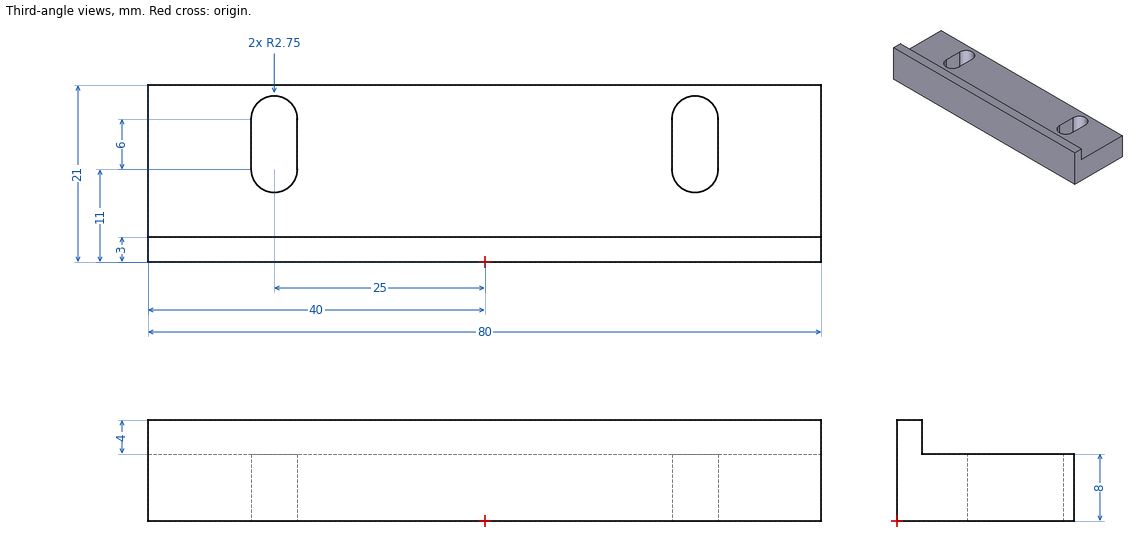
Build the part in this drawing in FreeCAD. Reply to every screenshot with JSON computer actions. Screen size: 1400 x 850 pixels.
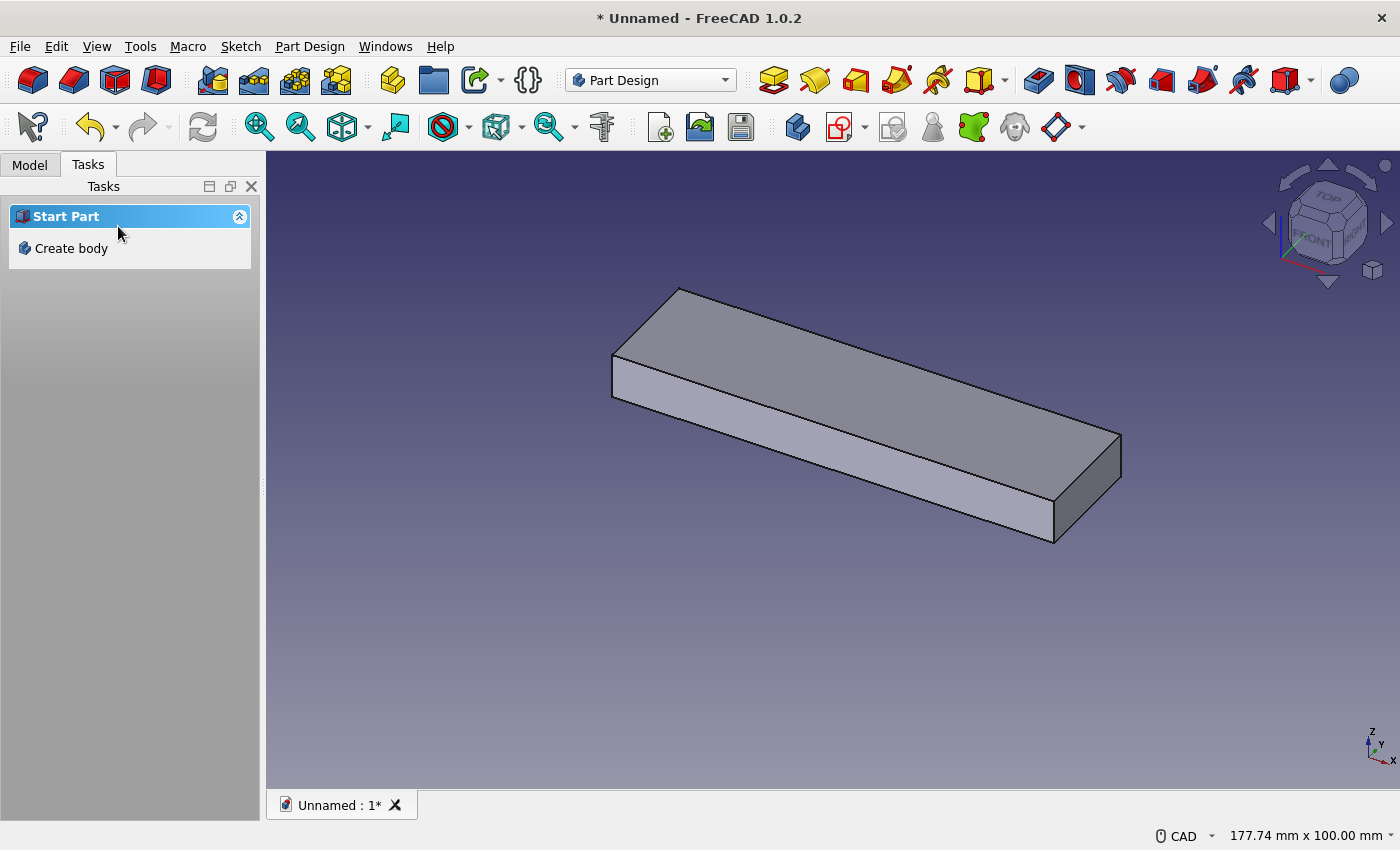
{"action": "key", "text": "v f"}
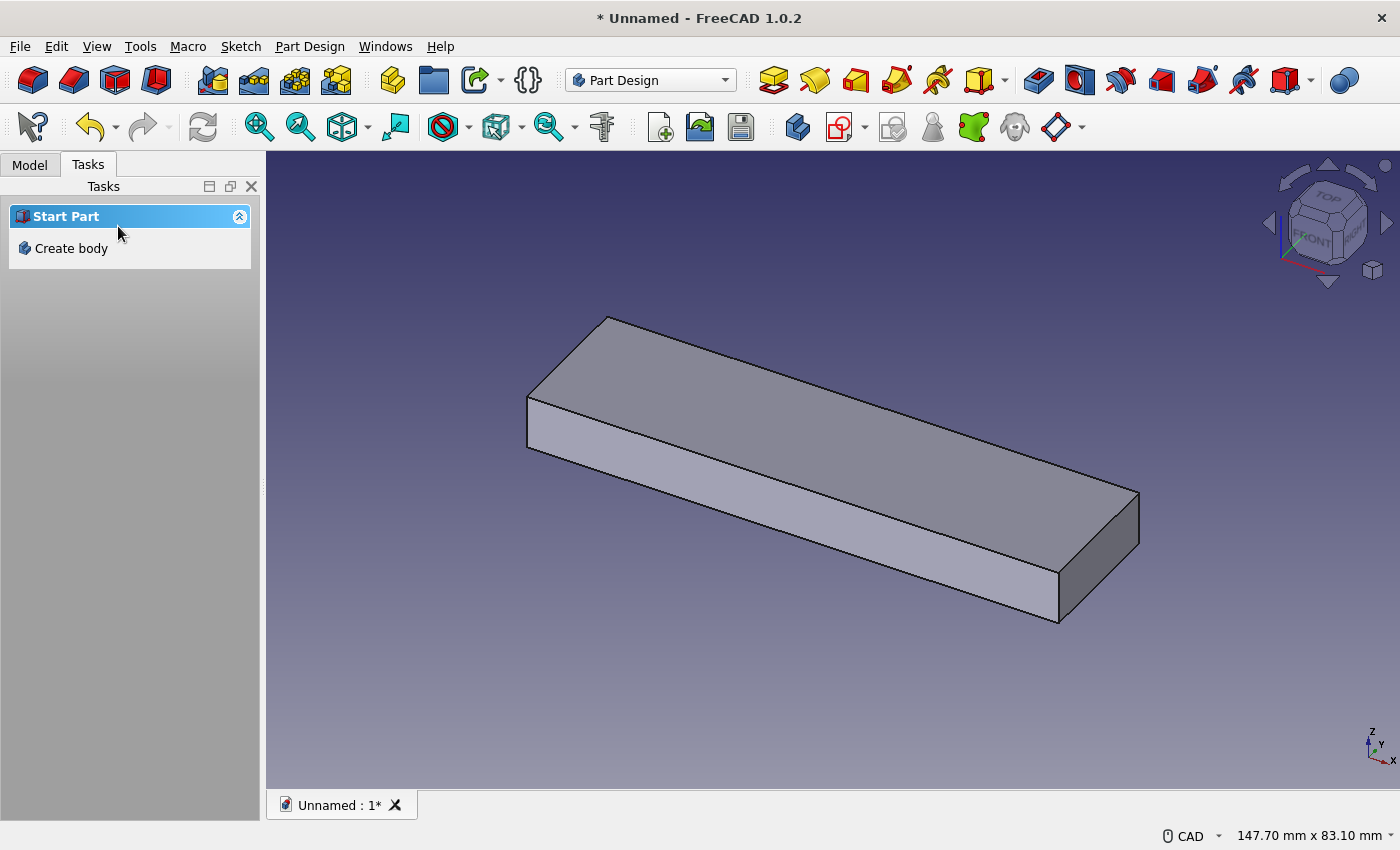
{"action": "left_click", "coordinate": [985, 494]}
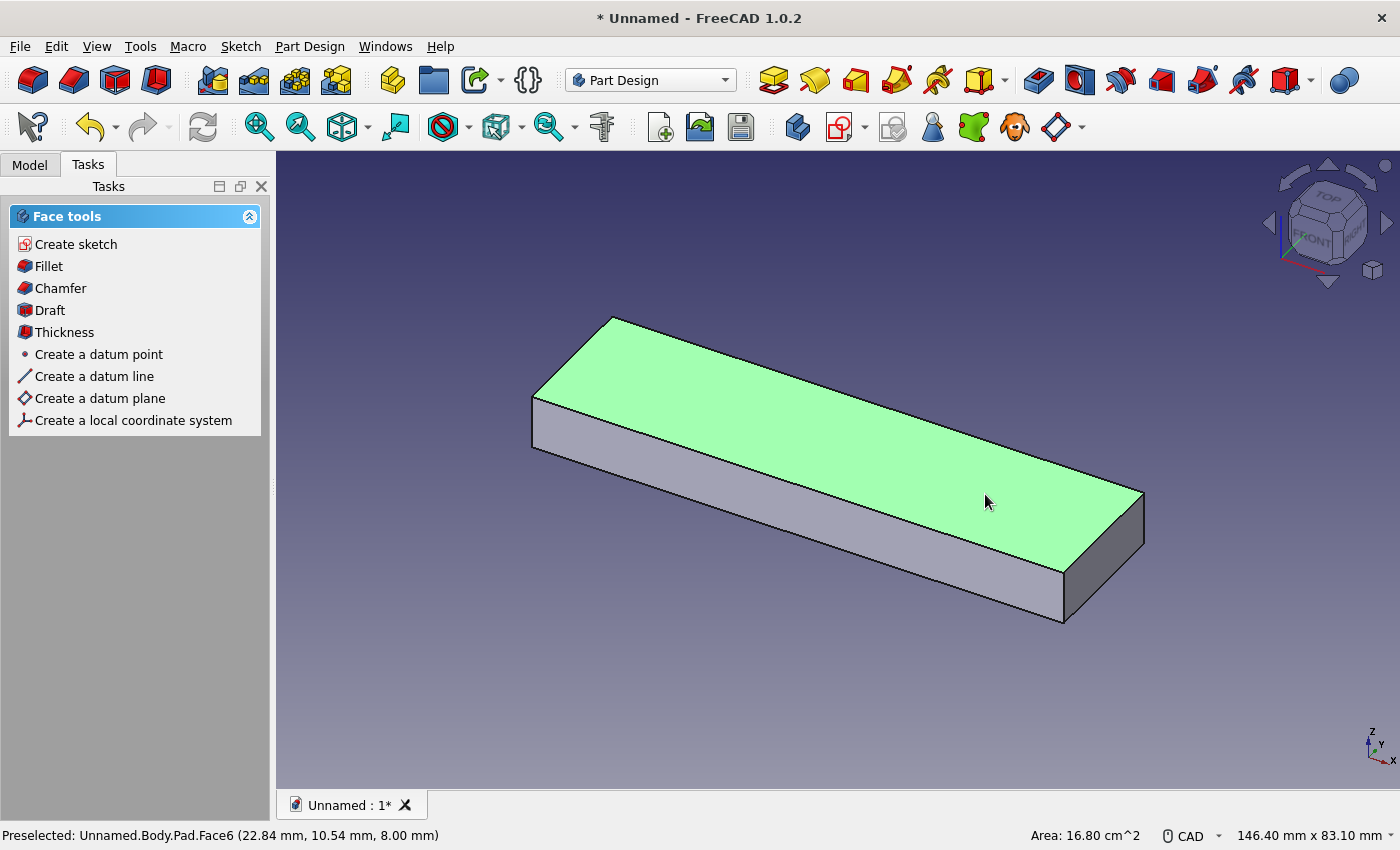
{"action": "left_click", "coordinate": [838, 128]}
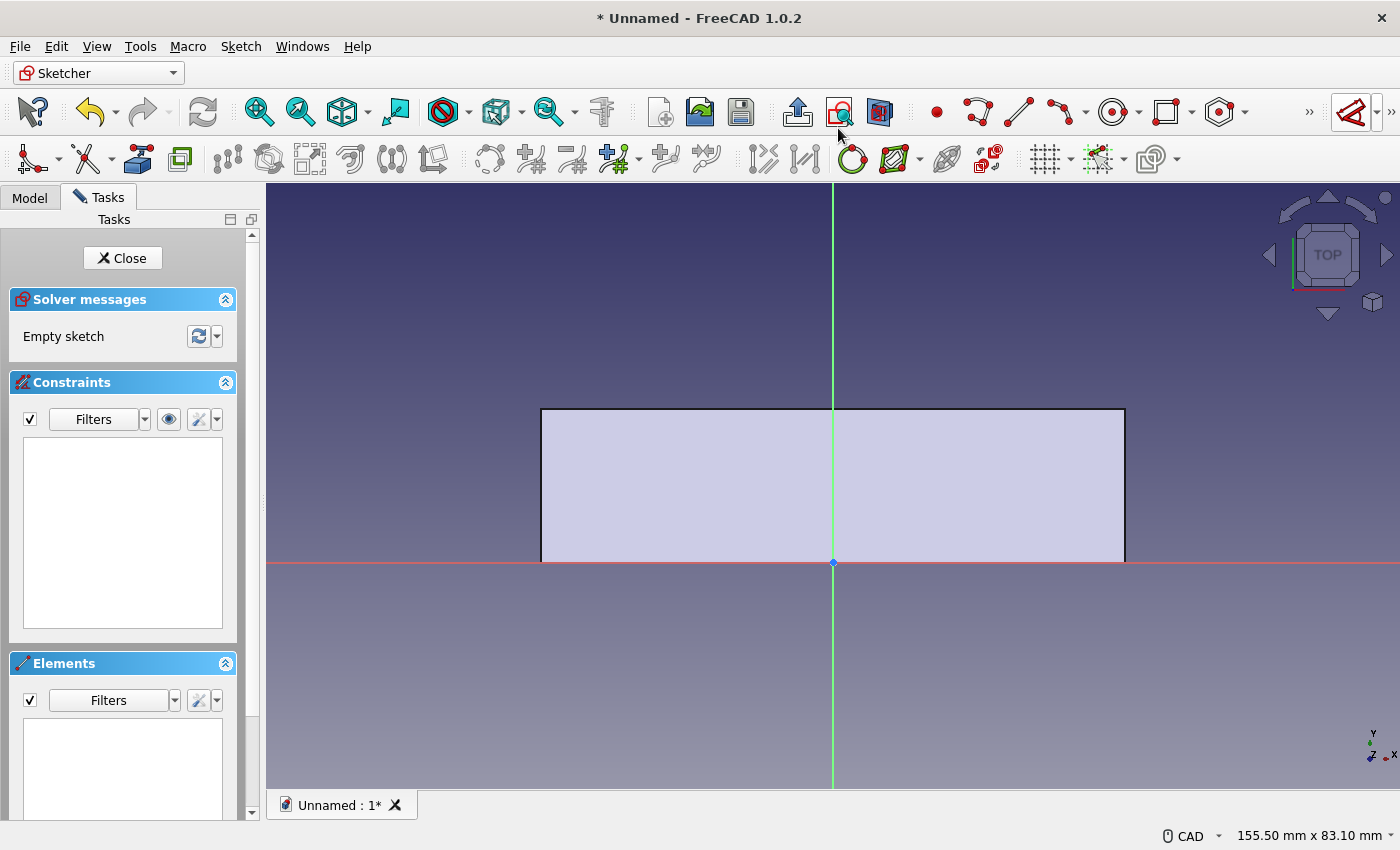
{"action": "left_click", "coordinate": [1166, 112]}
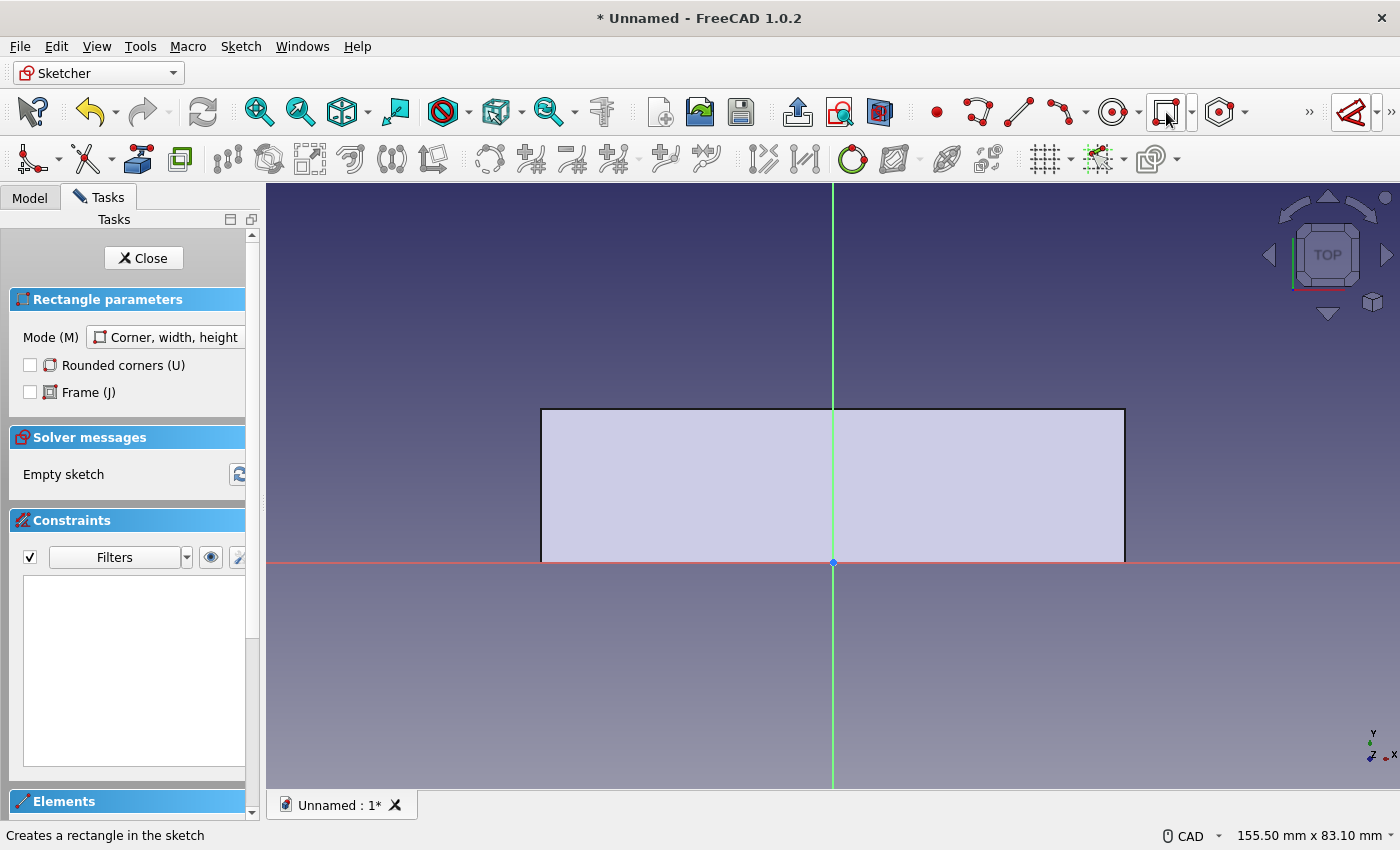
{"action": "left_click", "coordinate": [541, 541]}
{"action": "left_click", "coordinate": [1125, 563]}
{"action": "key", "text": "Escape"}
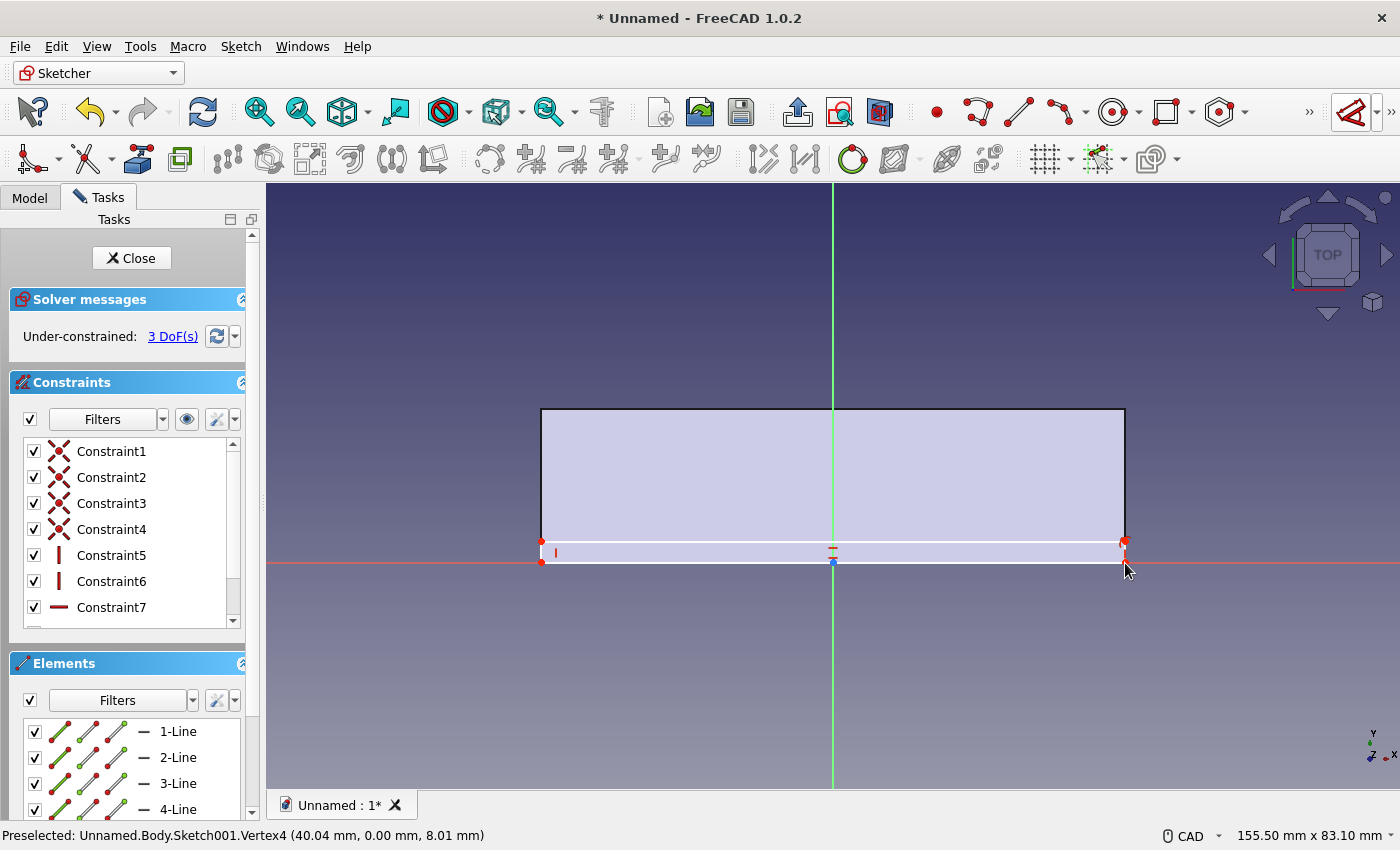
{"action": "left_click", "coordinate": [1350, 112]}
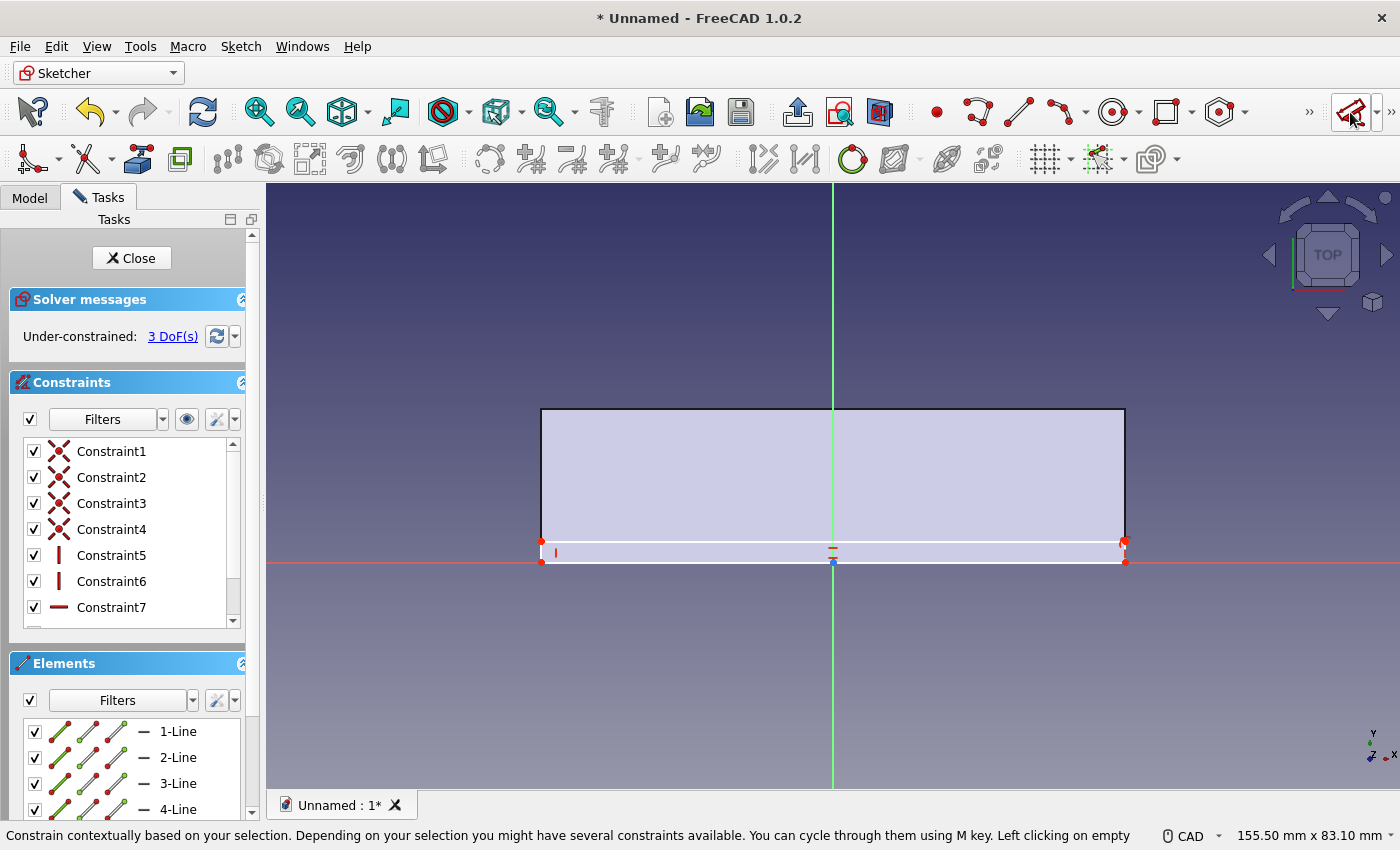
{"action": "scroll", "coordinate": [541, 552], "scroll_direction": "up", "scroll_amount": 3}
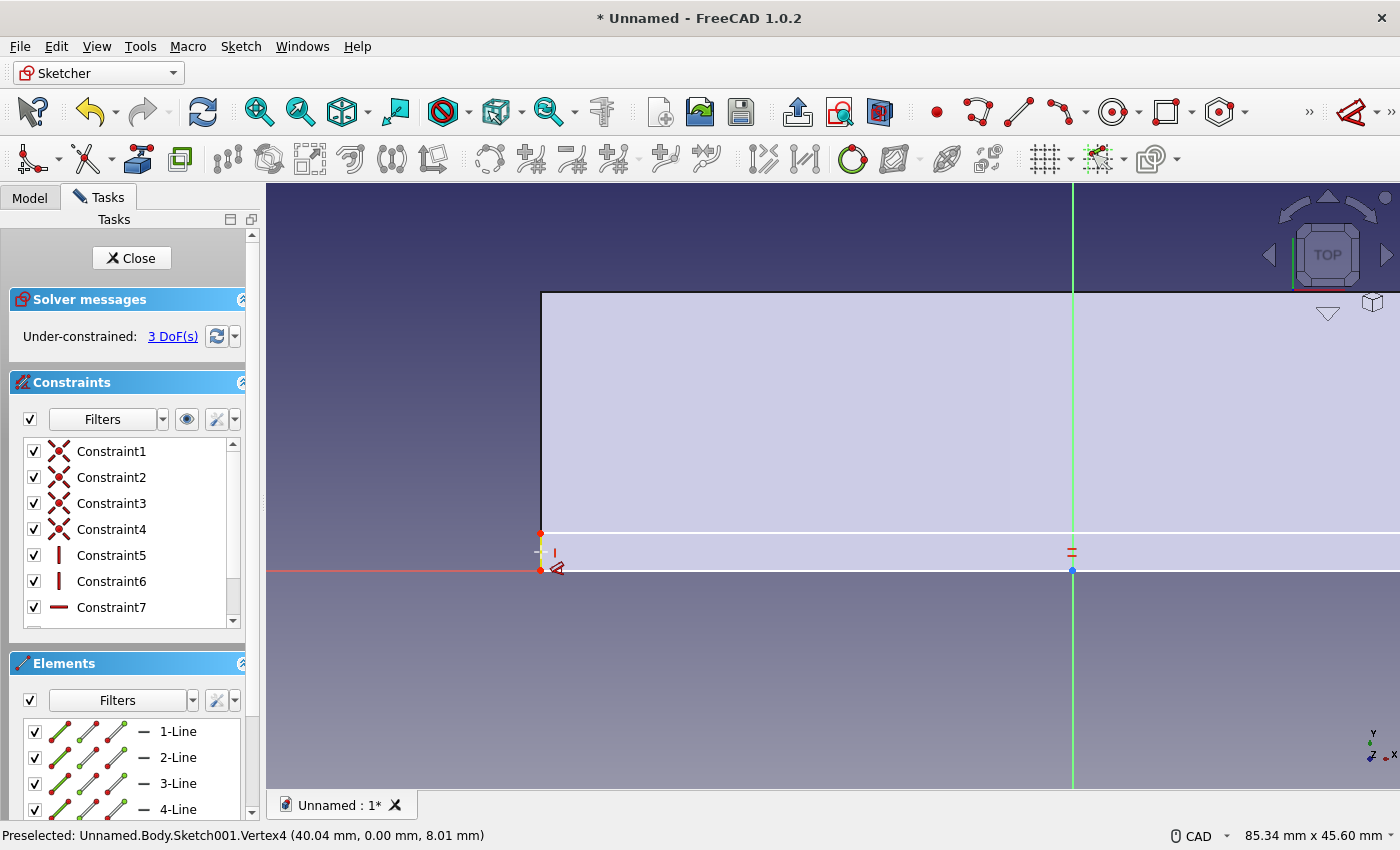
{"action": "left_click", "coordinate": [541, 552]}
{"action": "left_click", "coordinate": [507, 552]}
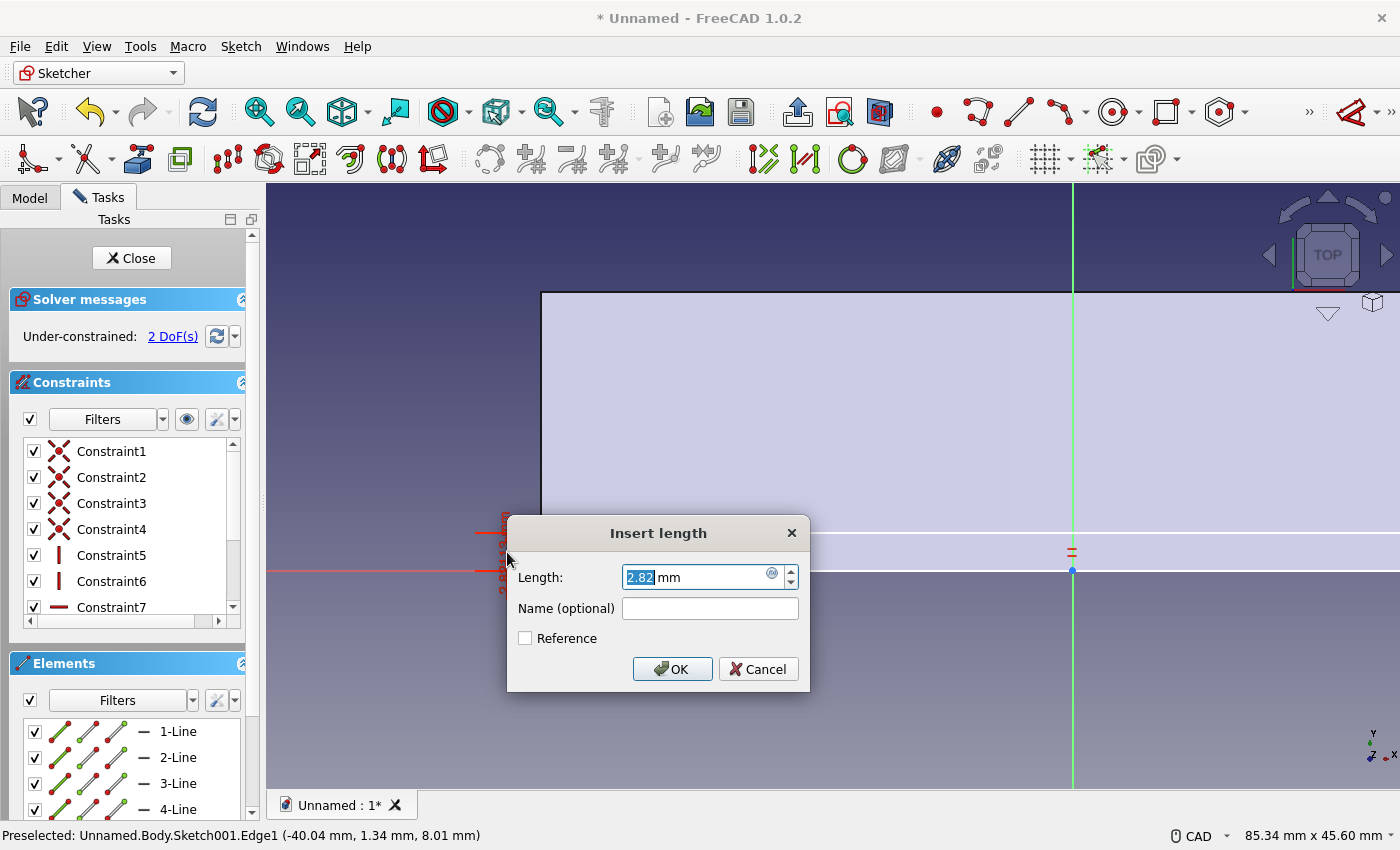
{"action": "type", "text": "3"}
{"action": "key", "text": "Return"}